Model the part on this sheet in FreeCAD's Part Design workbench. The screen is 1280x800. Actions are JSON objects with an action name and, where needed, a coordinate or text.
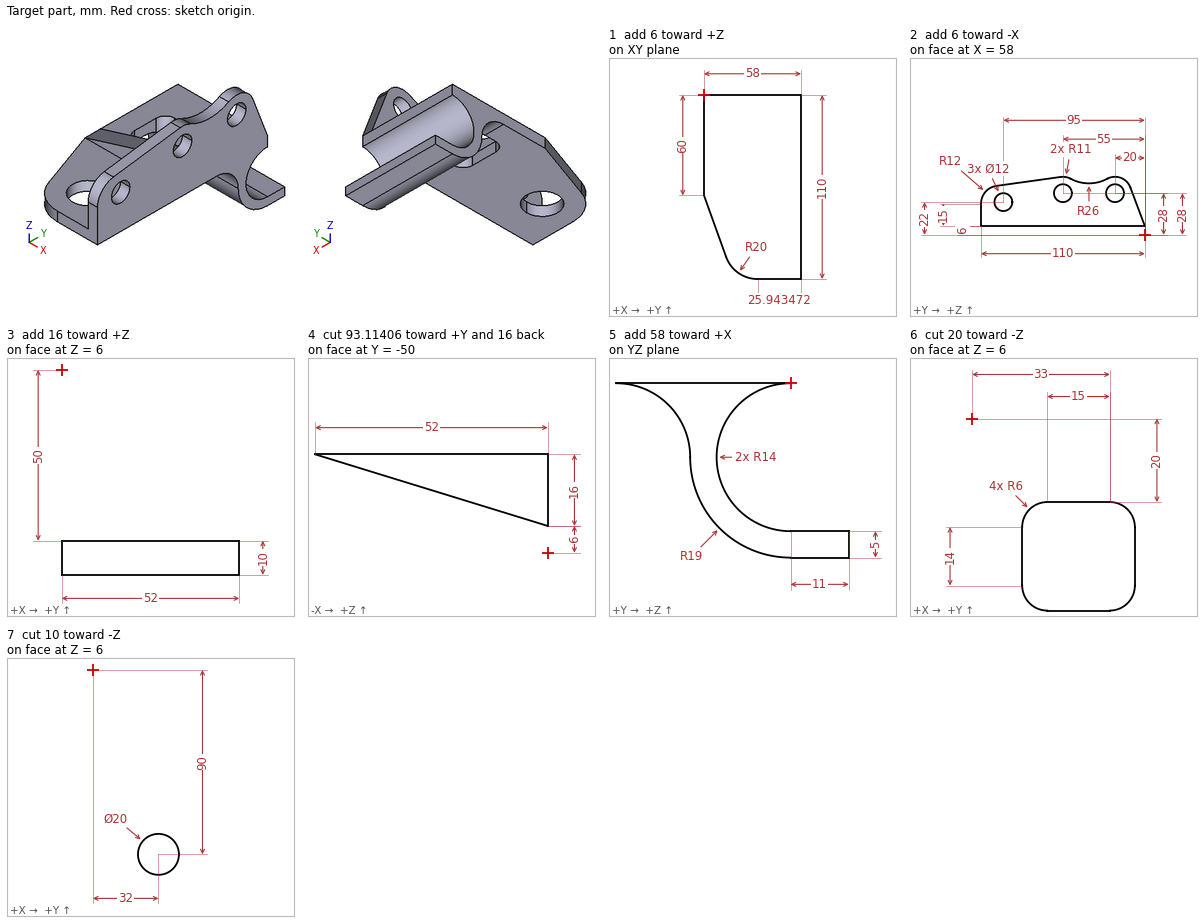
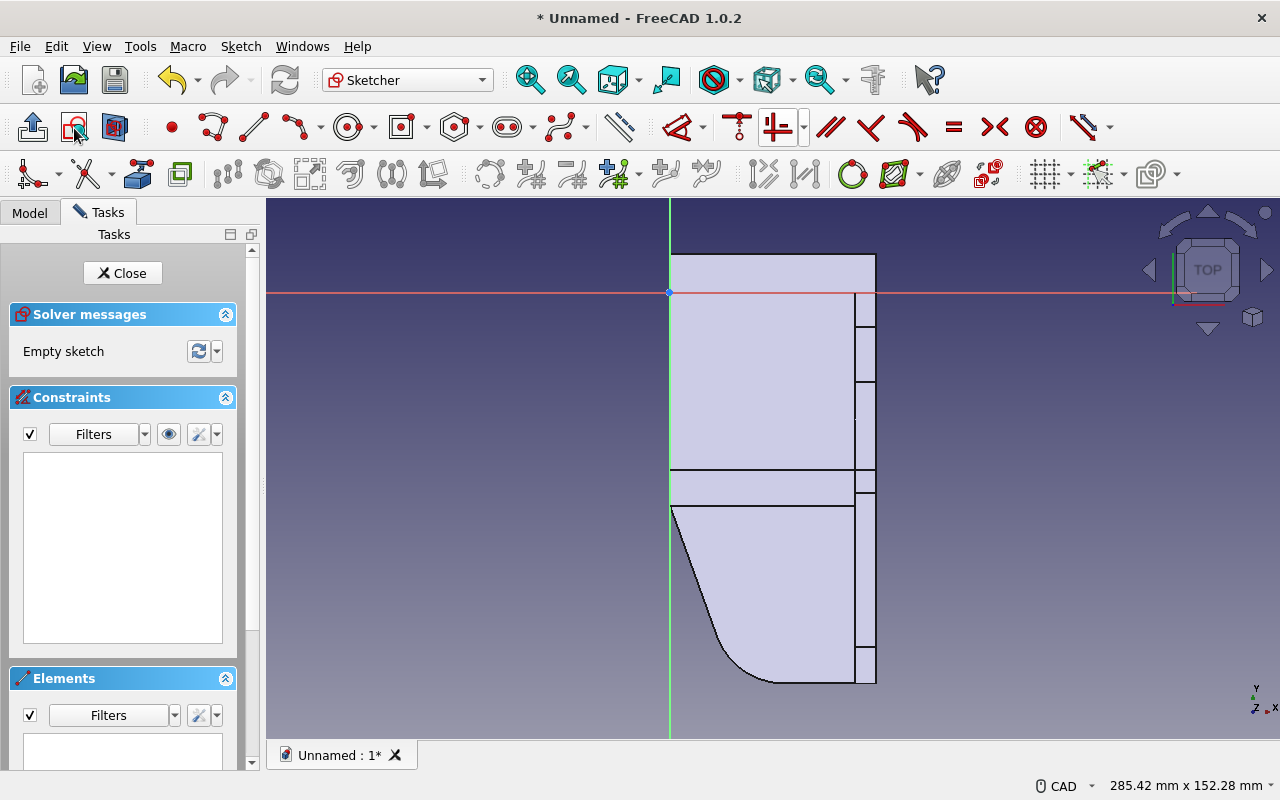
{"action": "scroll", "coordinate": [768, 298], "scroll_direction": "up", "scroll_amount": 4}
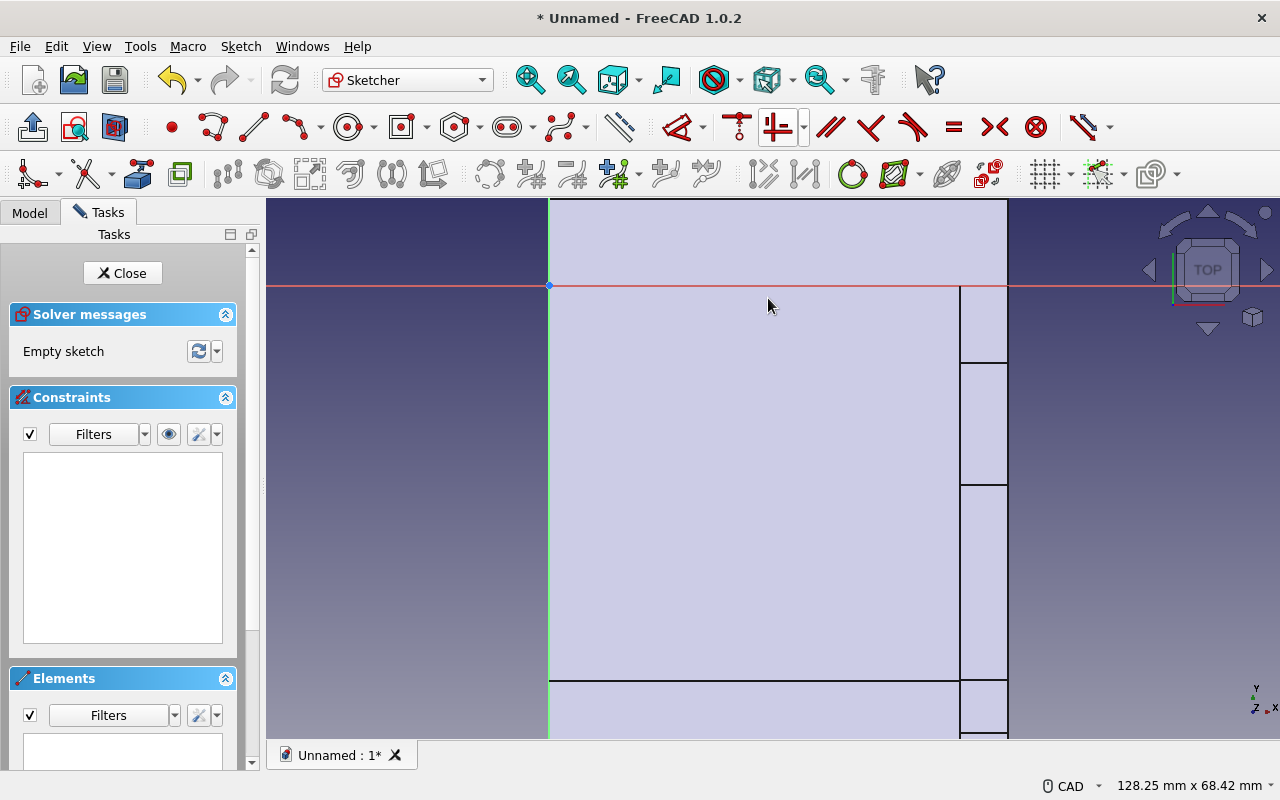
{"action": "left_click", "coordinate": [254, 128]}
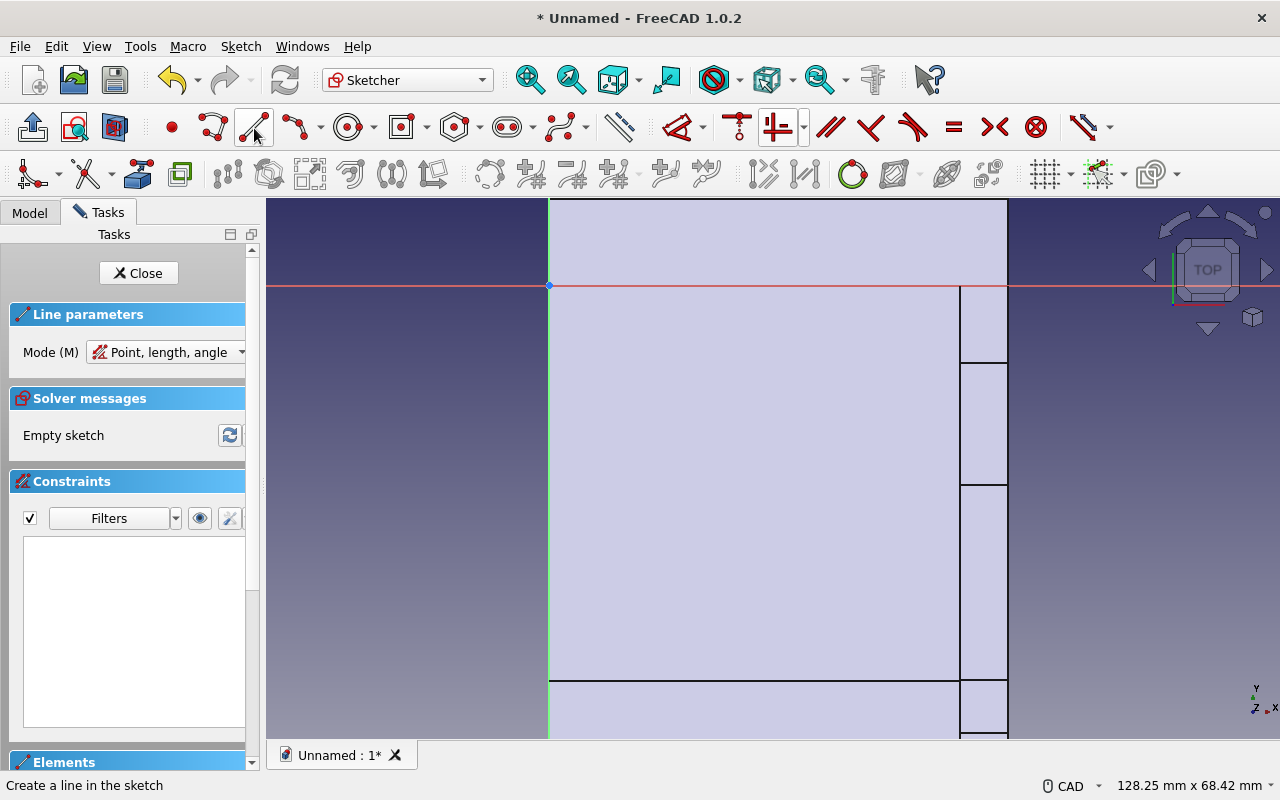
{"action": "left_click", "coordinate": [810, 444]}
{"action": "left_click", "coordinate": [692, 444]}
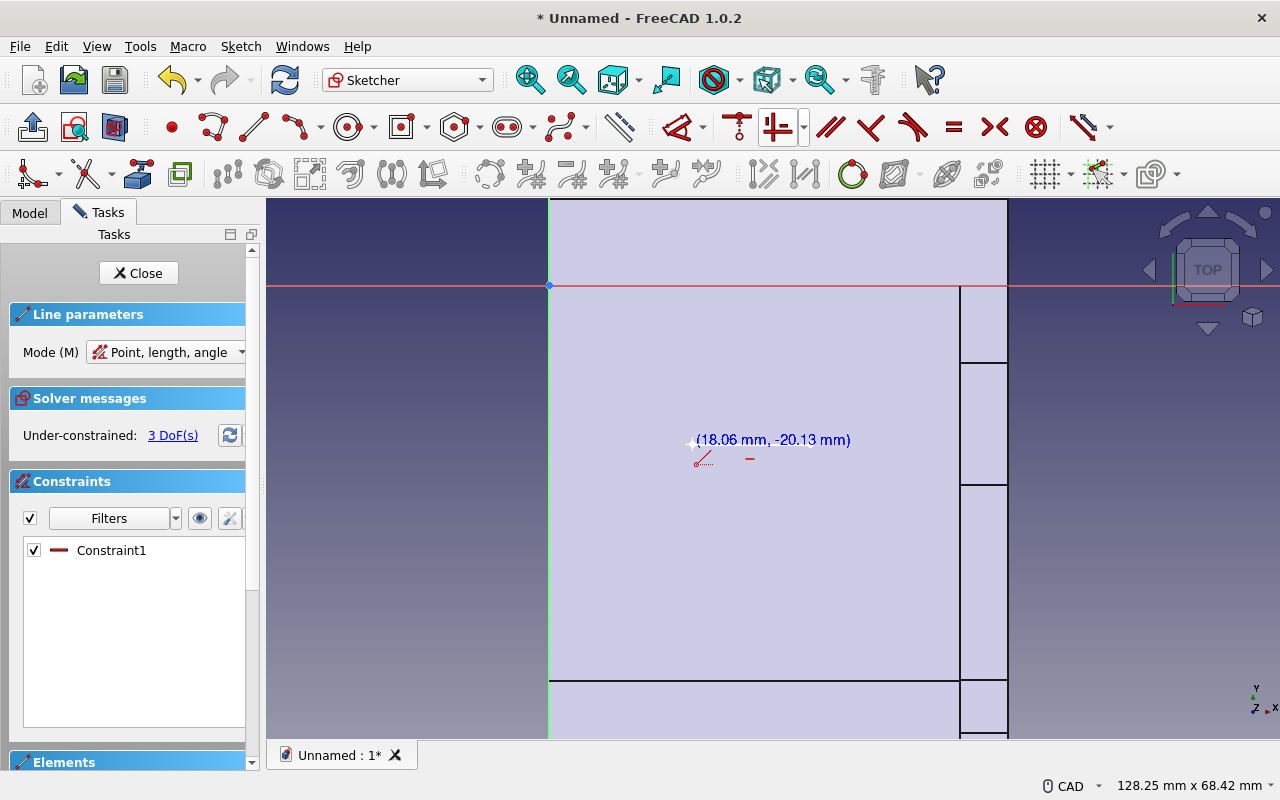
{"action": "left_click", "coordinate": [644, 491]}
{"action": "left_click", "coordinate": [644, 602]}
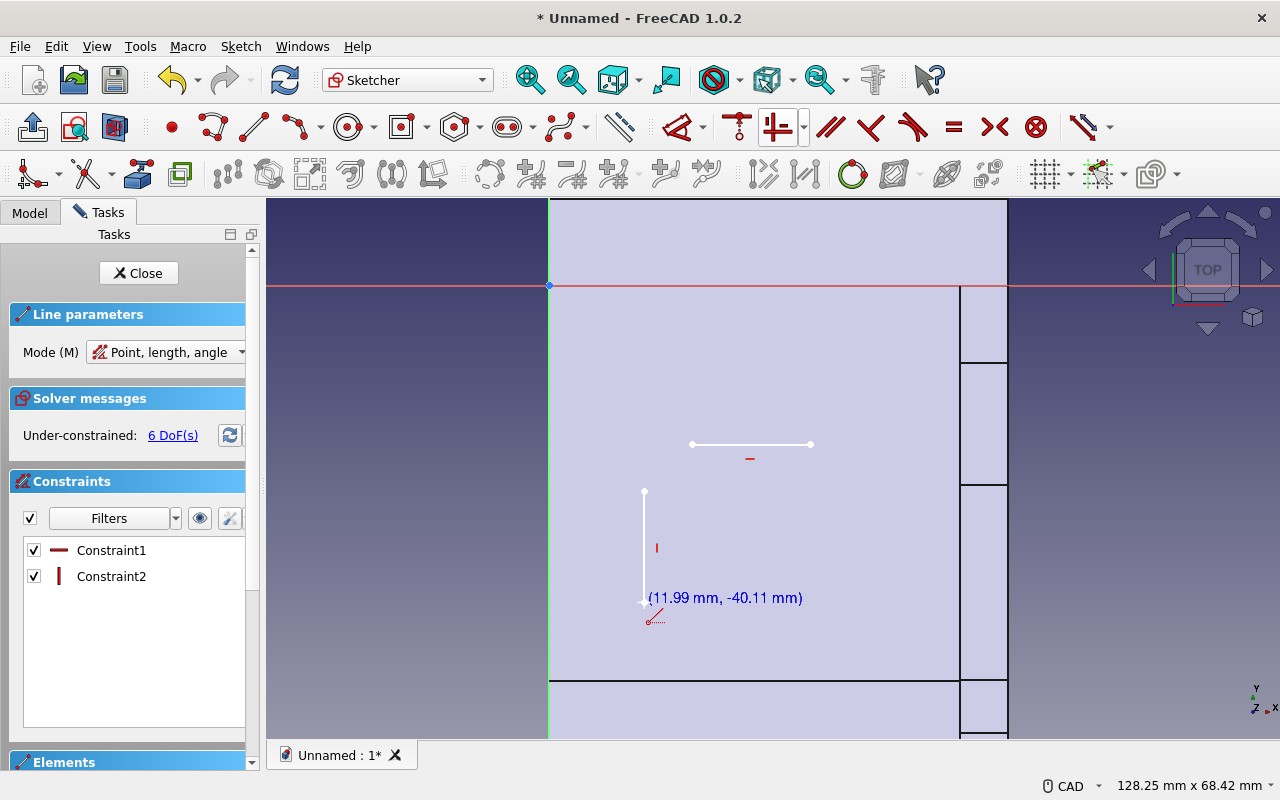
{"action": "left_click", "coordinate": [692, 650]}
{"action": "left_click", "coordinate": [810, 650]}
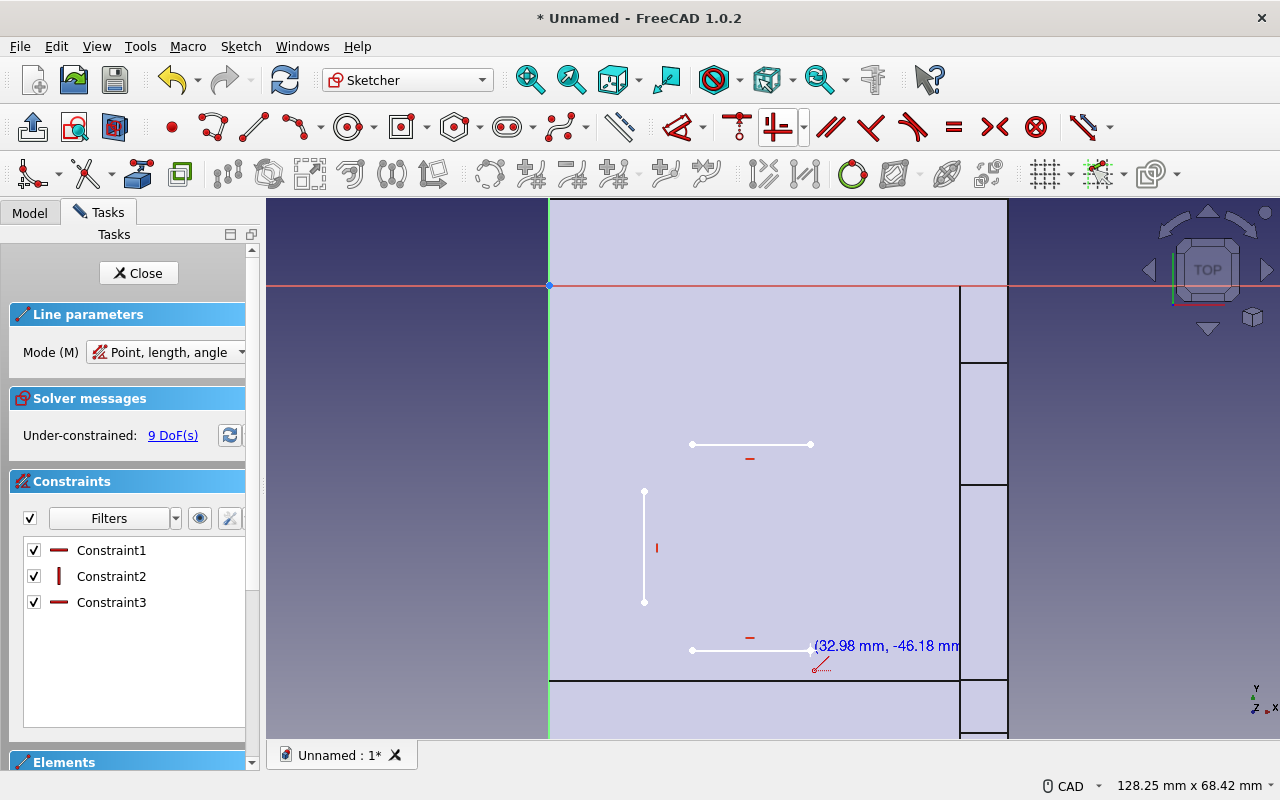
{"action": "left_click", "coordinate": [858, 602]}
{"action": "left_click", "coordinate": [858, 491]}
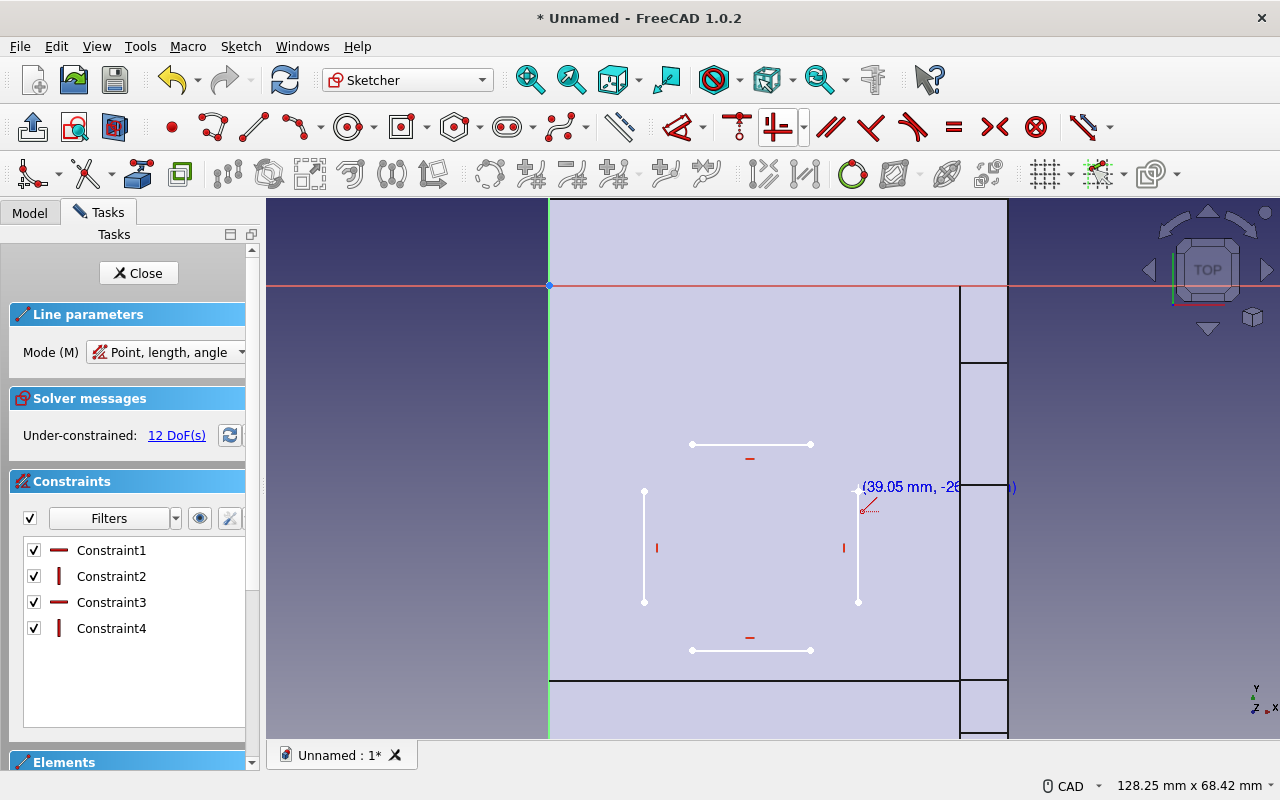
{"action": "left_click", "coordinate": [294, 128]}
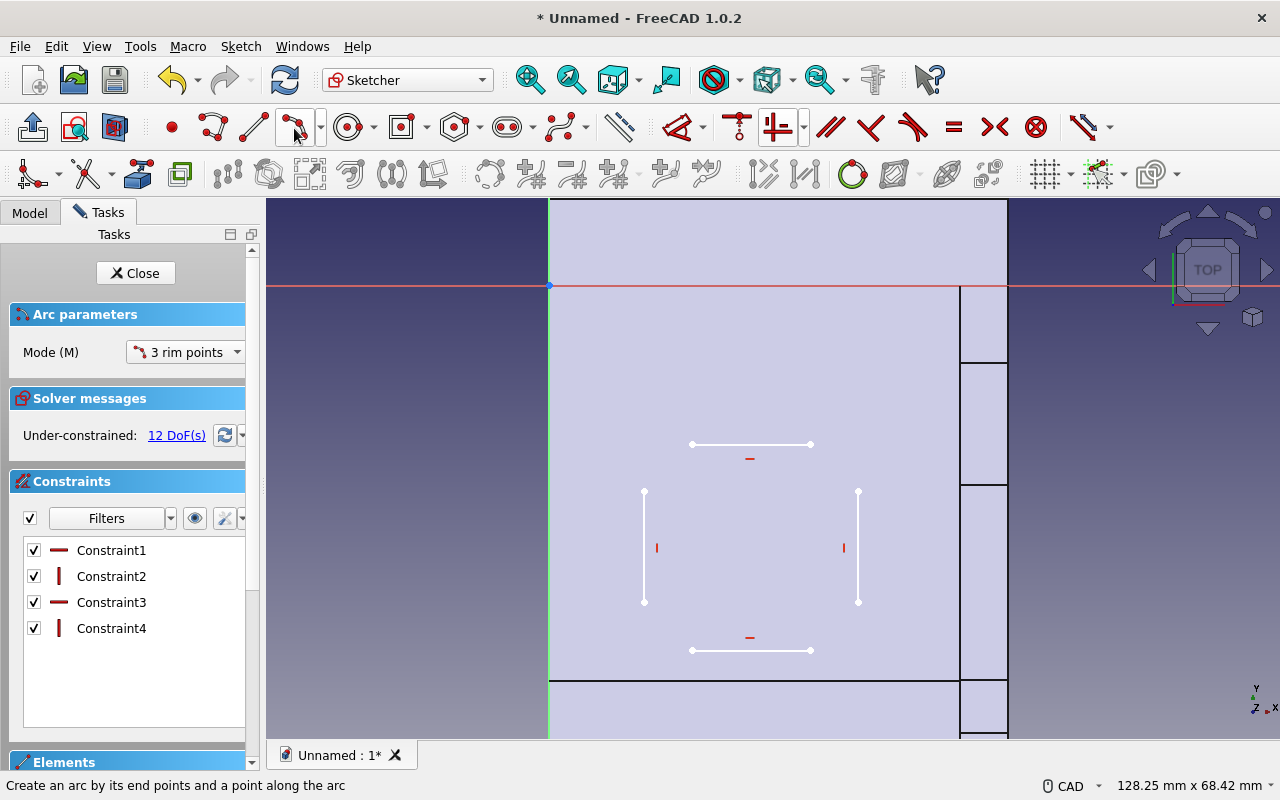
{"action": "left_click", "coordinate": [692, 445]}
{"action": "left_click", "coordinate": [644, 492]}
{"action": "left_click", "coordinate": [658, 458]}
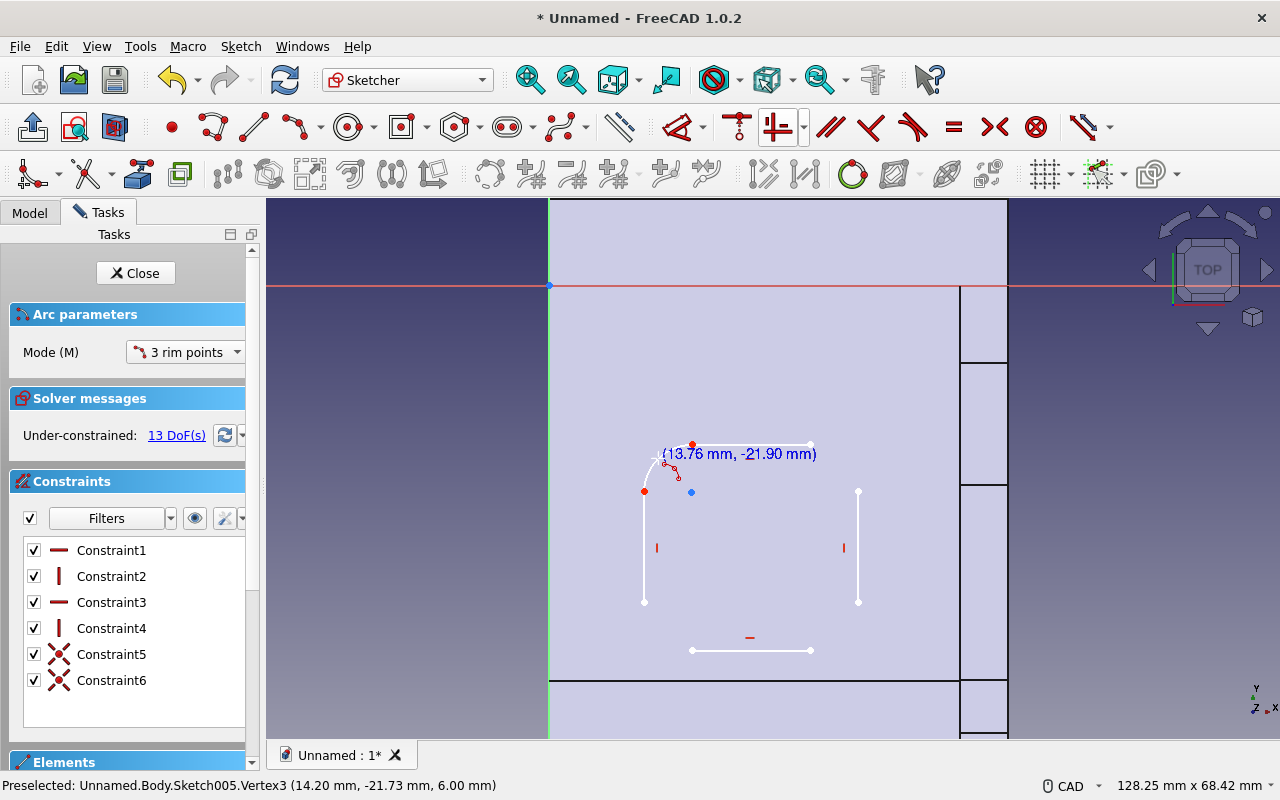
{"action": "left_click", "coordinate": [644, 603]}
{"action": "left_click", "coordinate": [692, 651]}
{"action": "left_click", "coordinate": [658, 636]}